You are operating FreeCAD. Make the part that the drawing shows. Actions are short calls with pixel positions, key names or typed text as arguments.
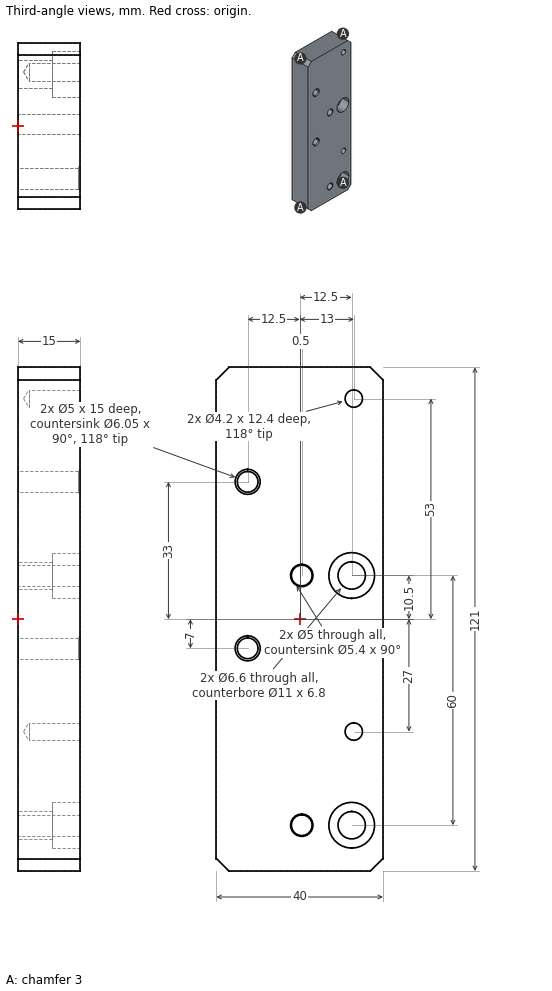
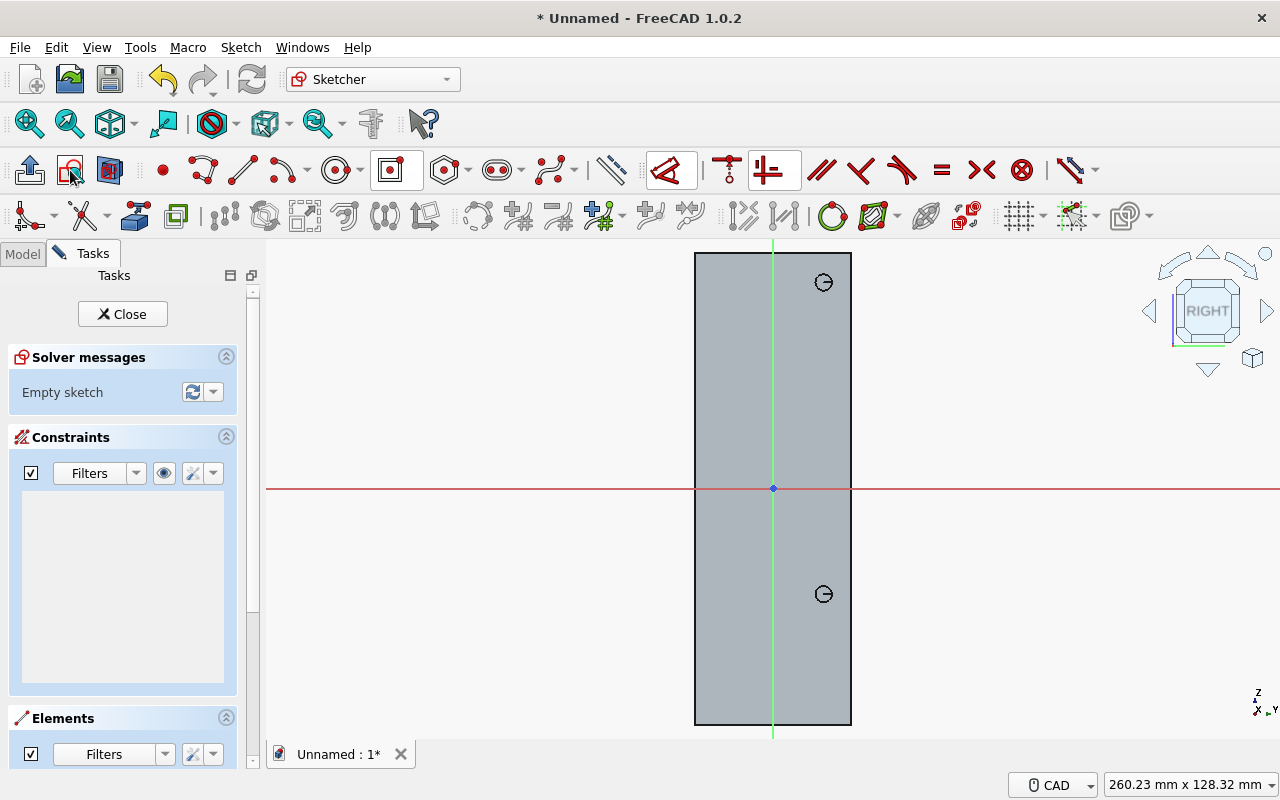
scroll(792, 377, up, 3)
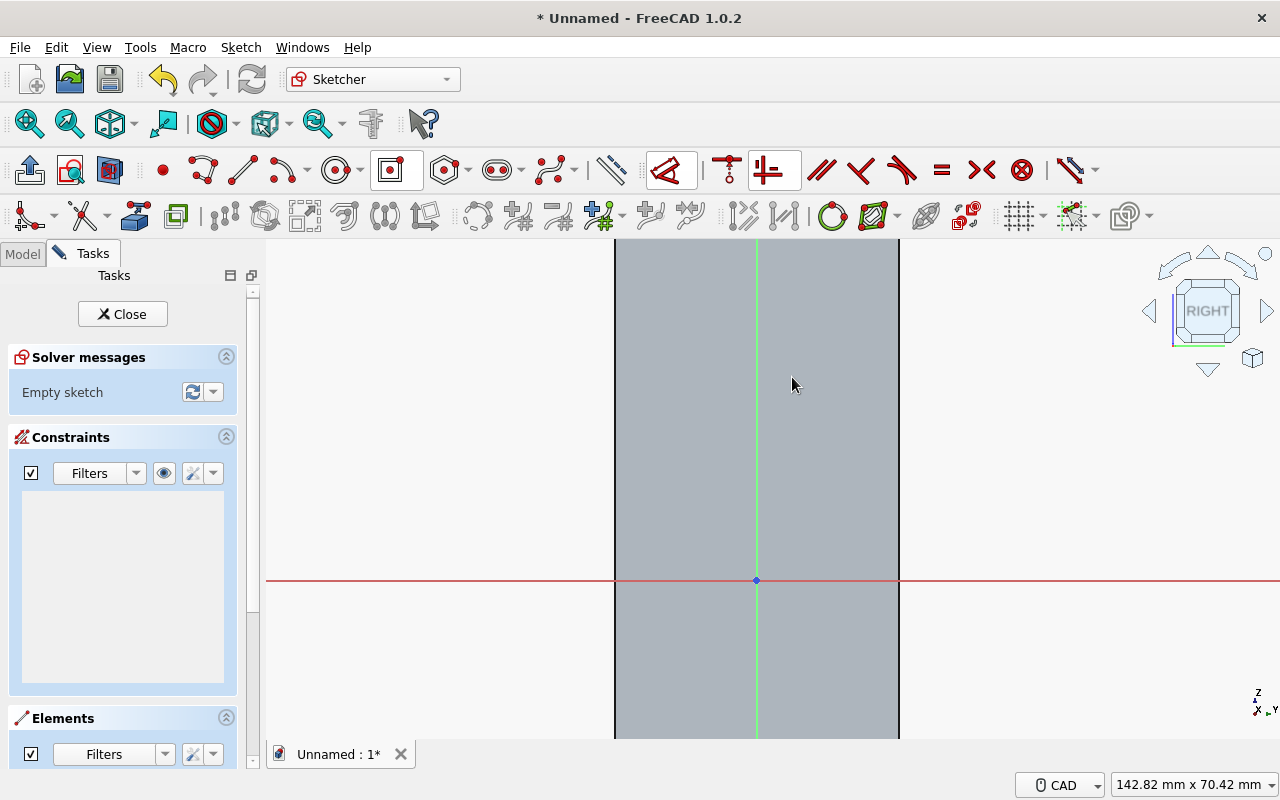
click(336, 170)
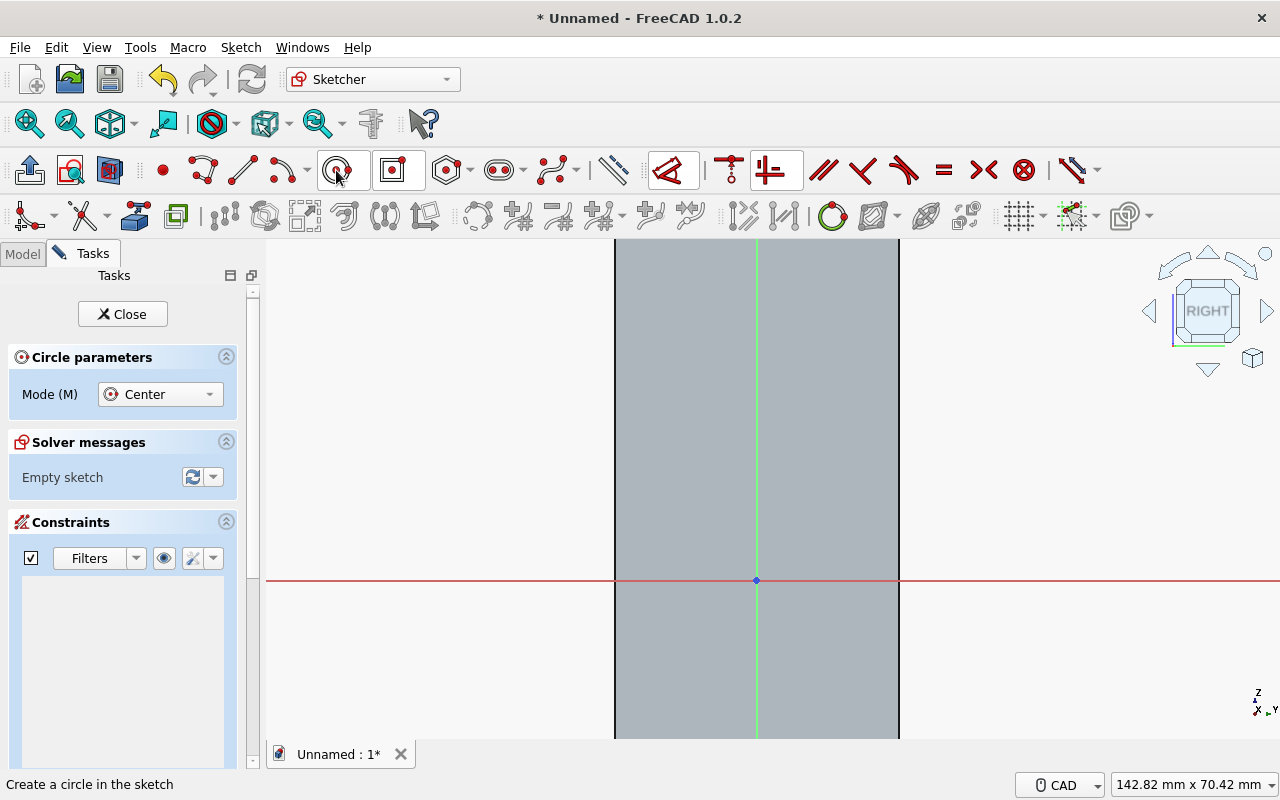
scroll(668, 347, up, 2)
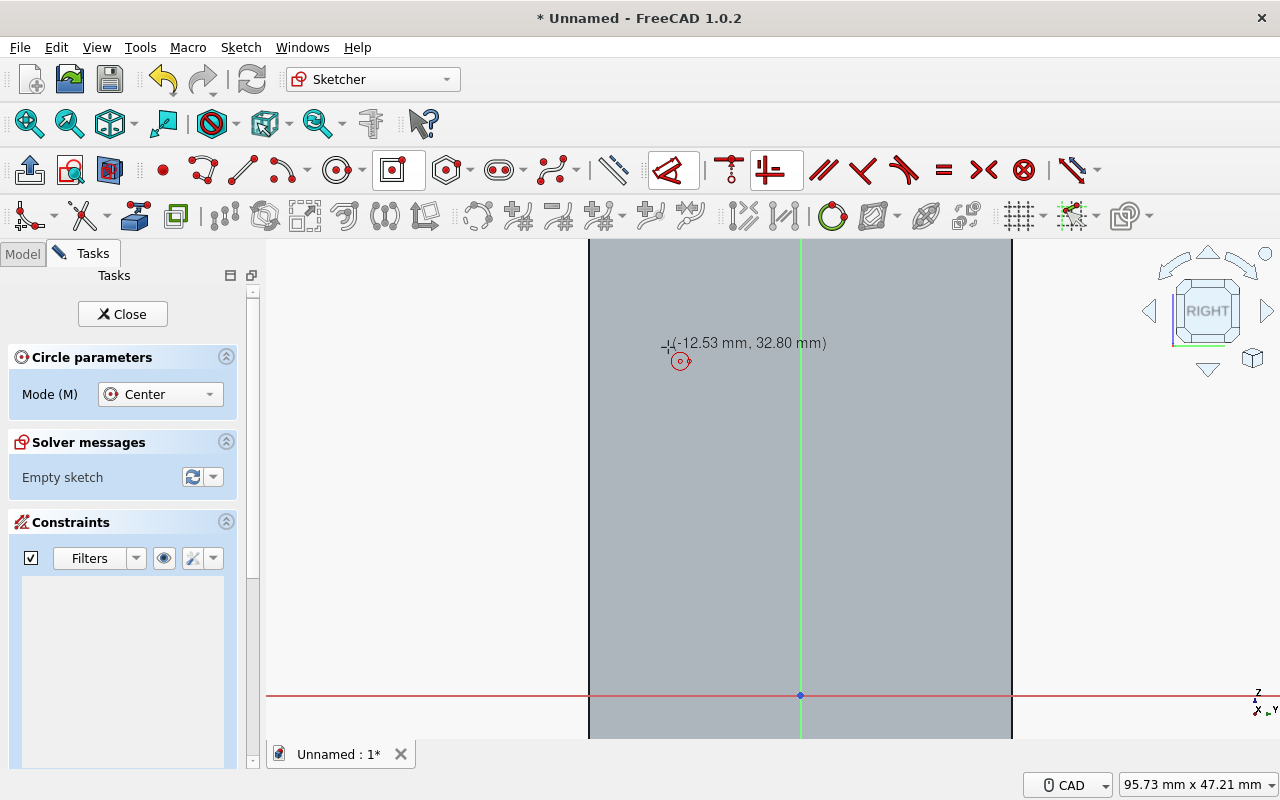
click(668, 346)
move(687, 328)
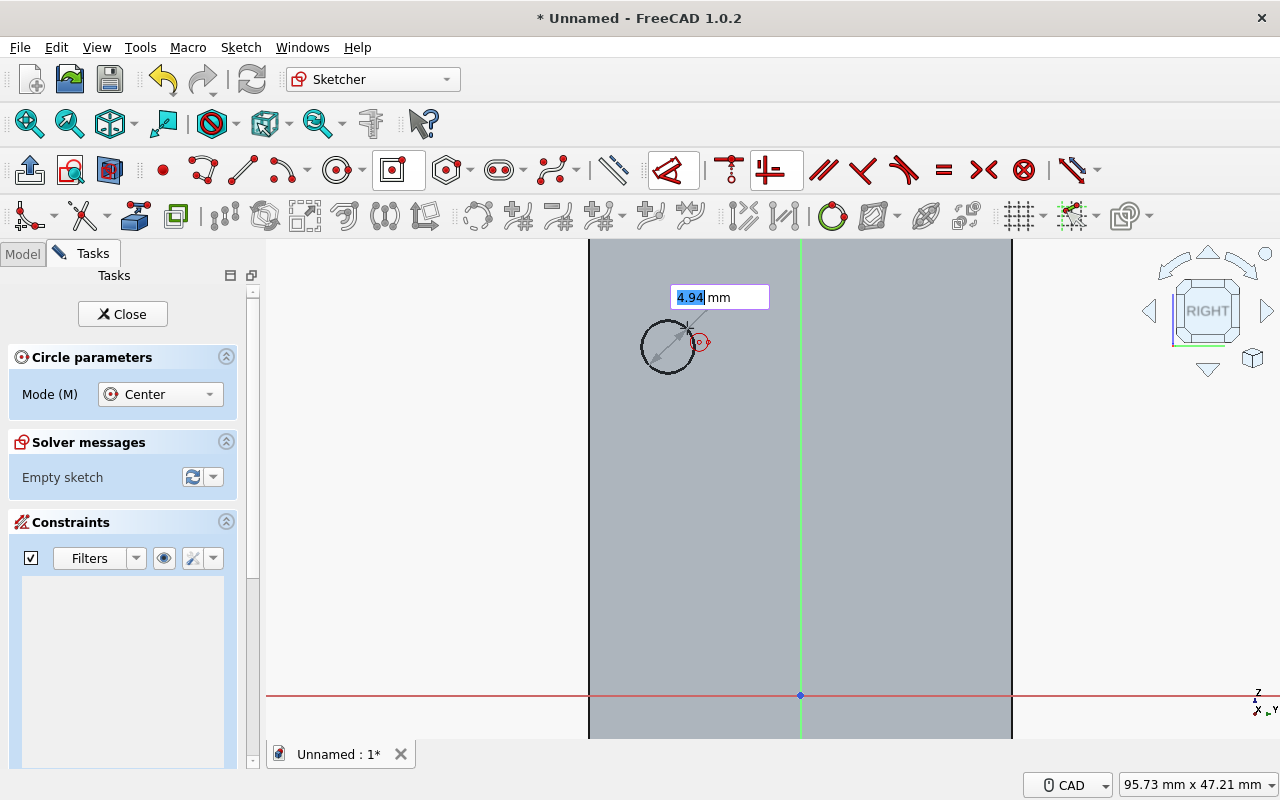
text(5)
key(Return)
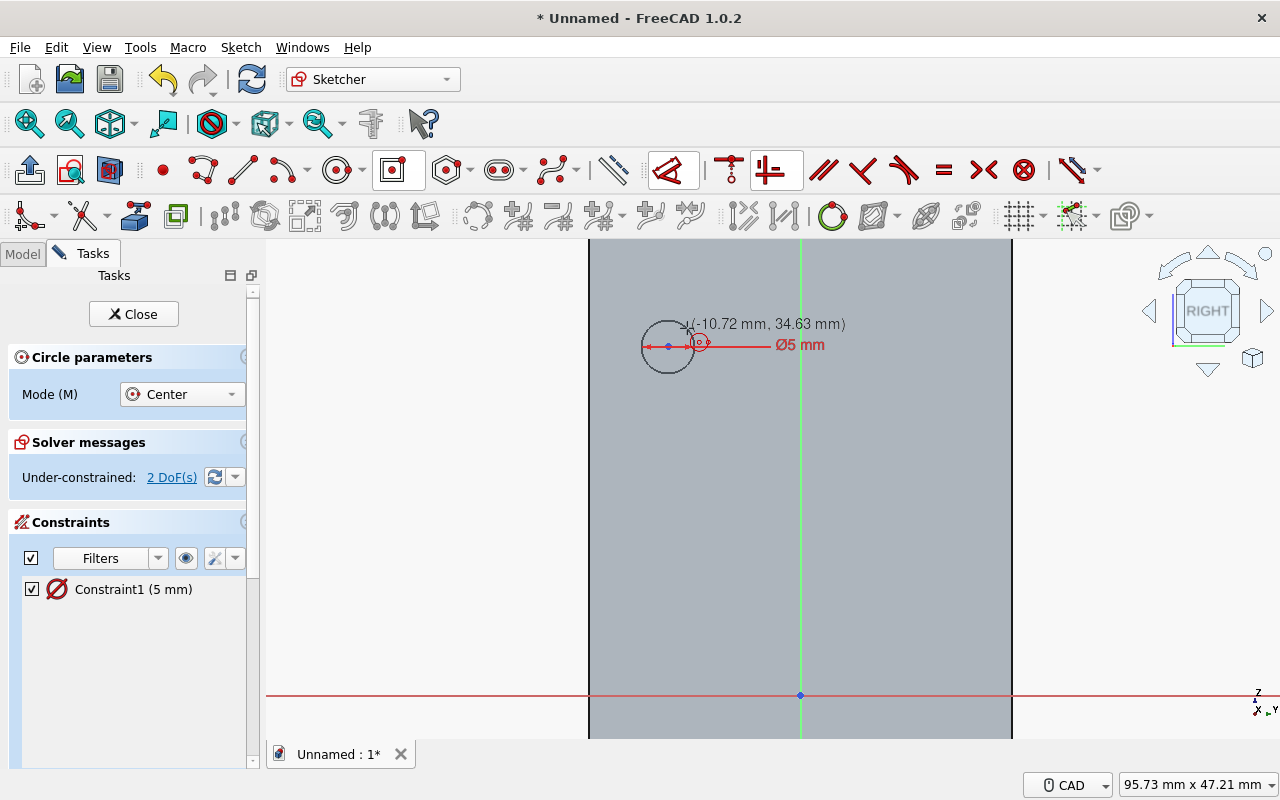
scroll(671, 349, down, 2)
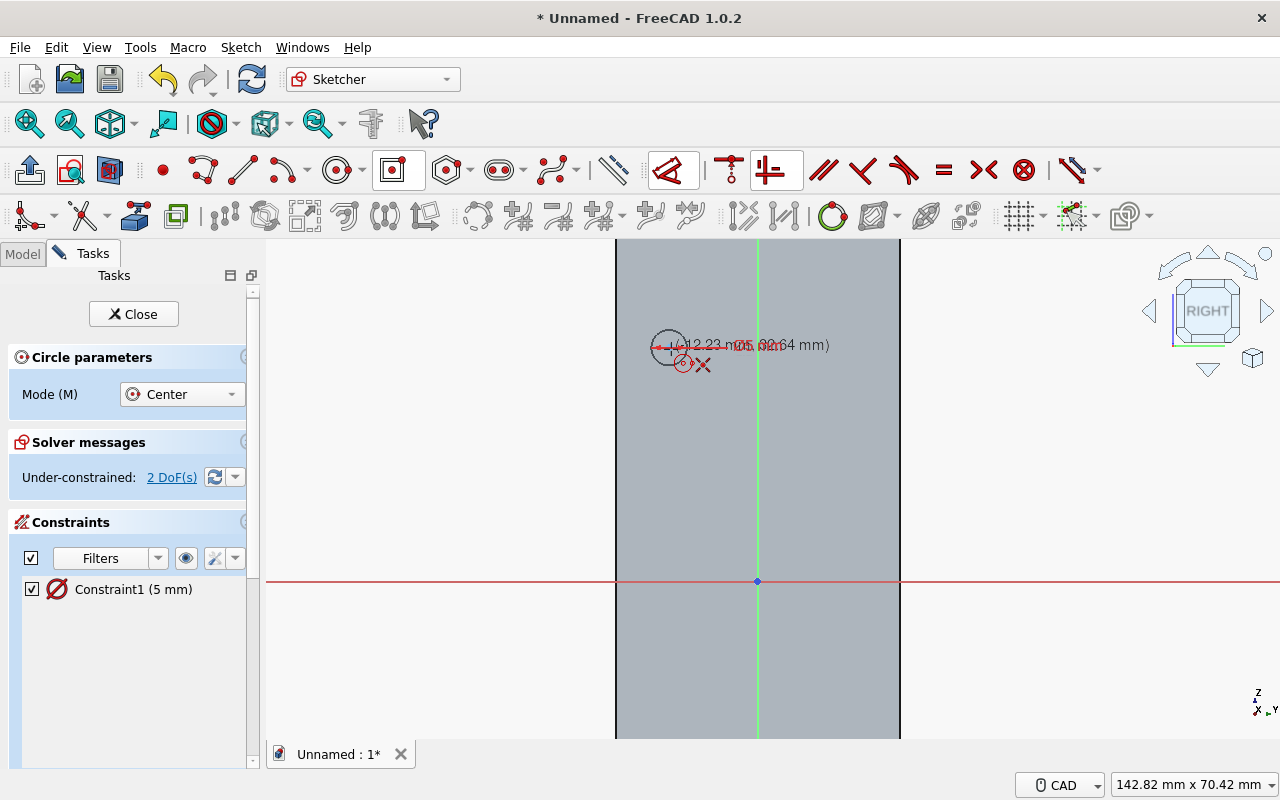
scroll(669, 631, up, 2)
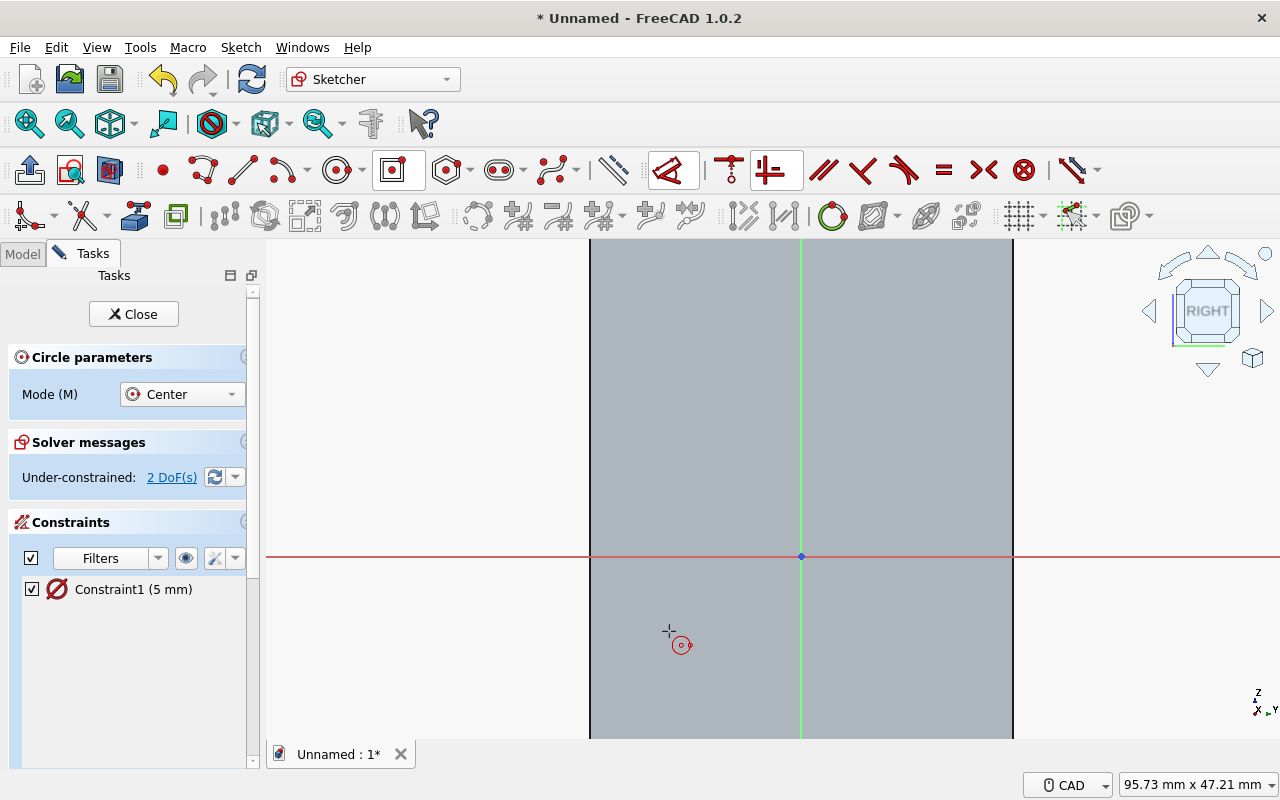
click(669, 631)
move(688, 612)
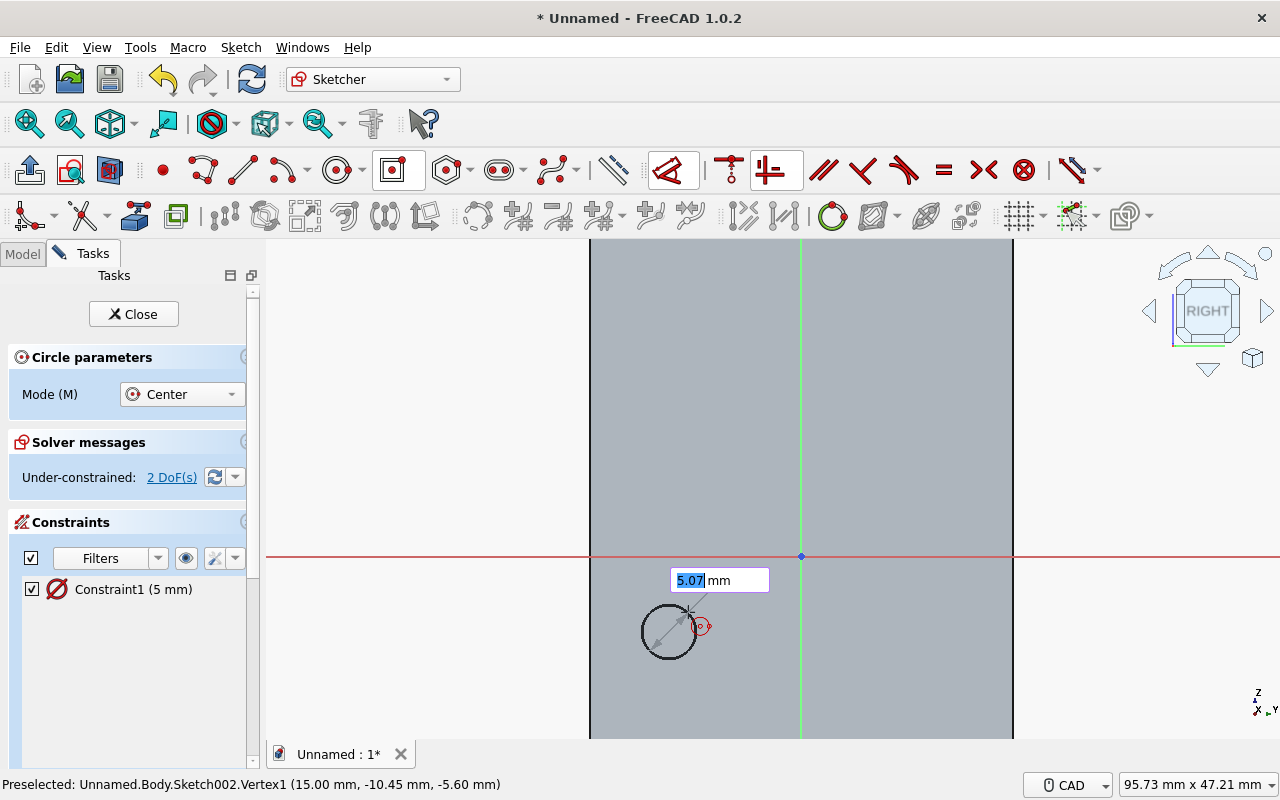
text(5)
key(Return)
key(Escape)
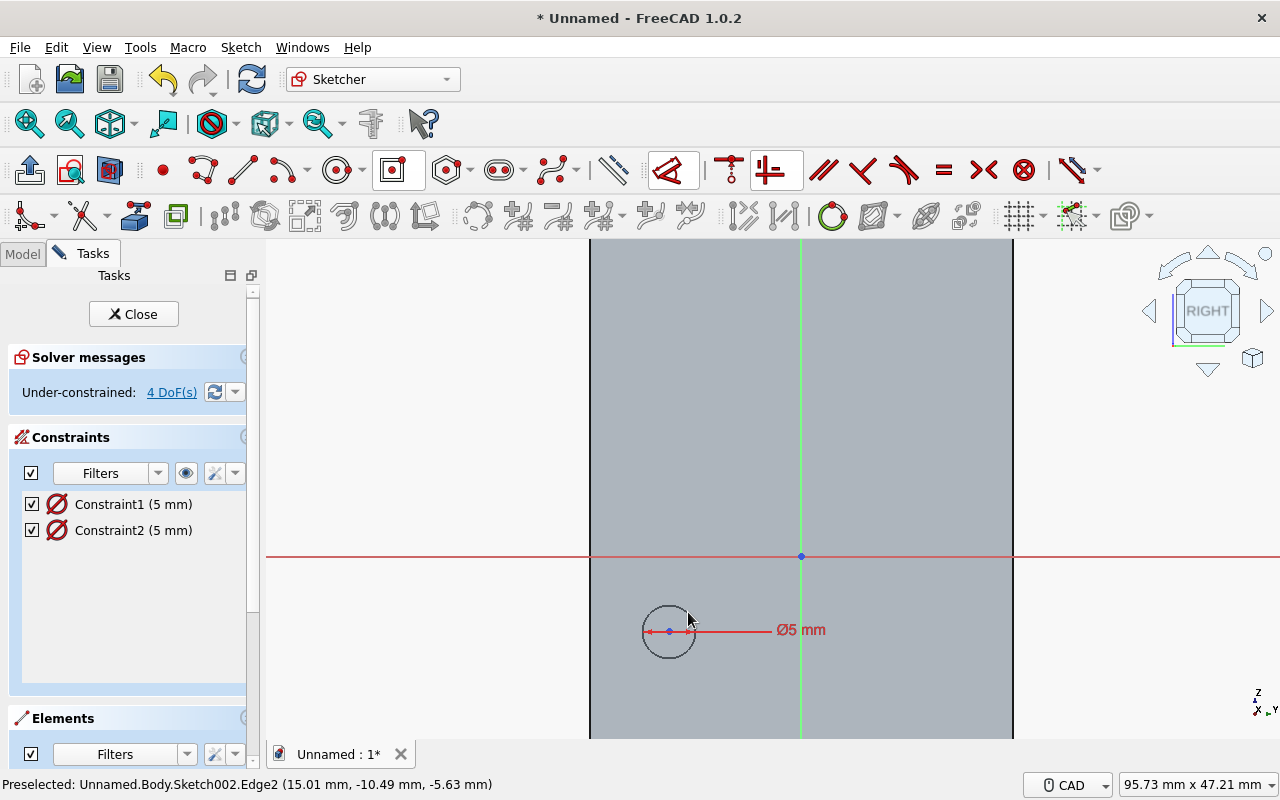
scroll(669, 631, down, 2)